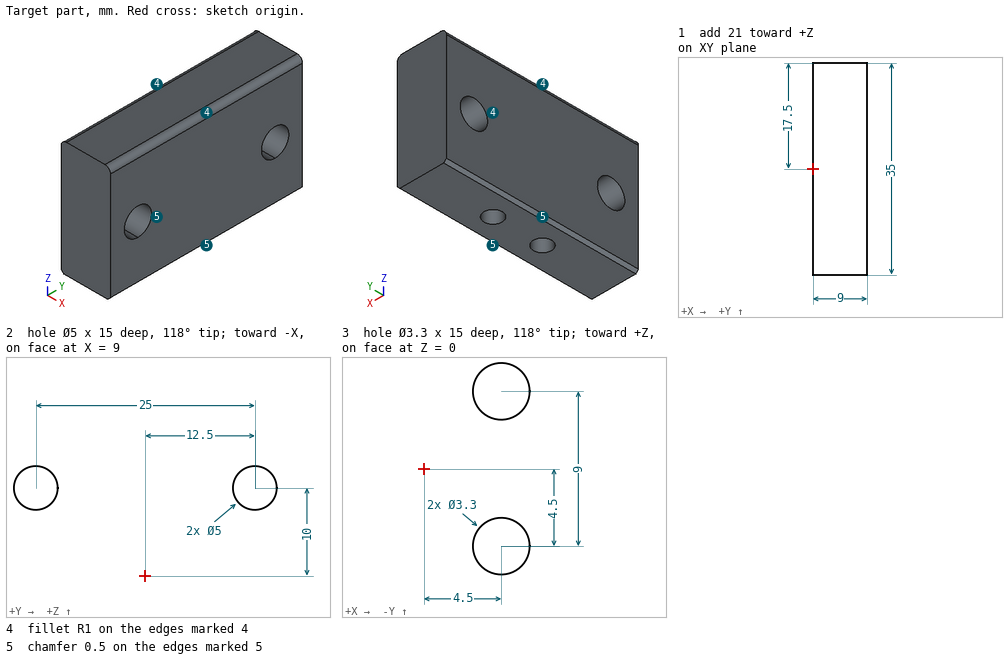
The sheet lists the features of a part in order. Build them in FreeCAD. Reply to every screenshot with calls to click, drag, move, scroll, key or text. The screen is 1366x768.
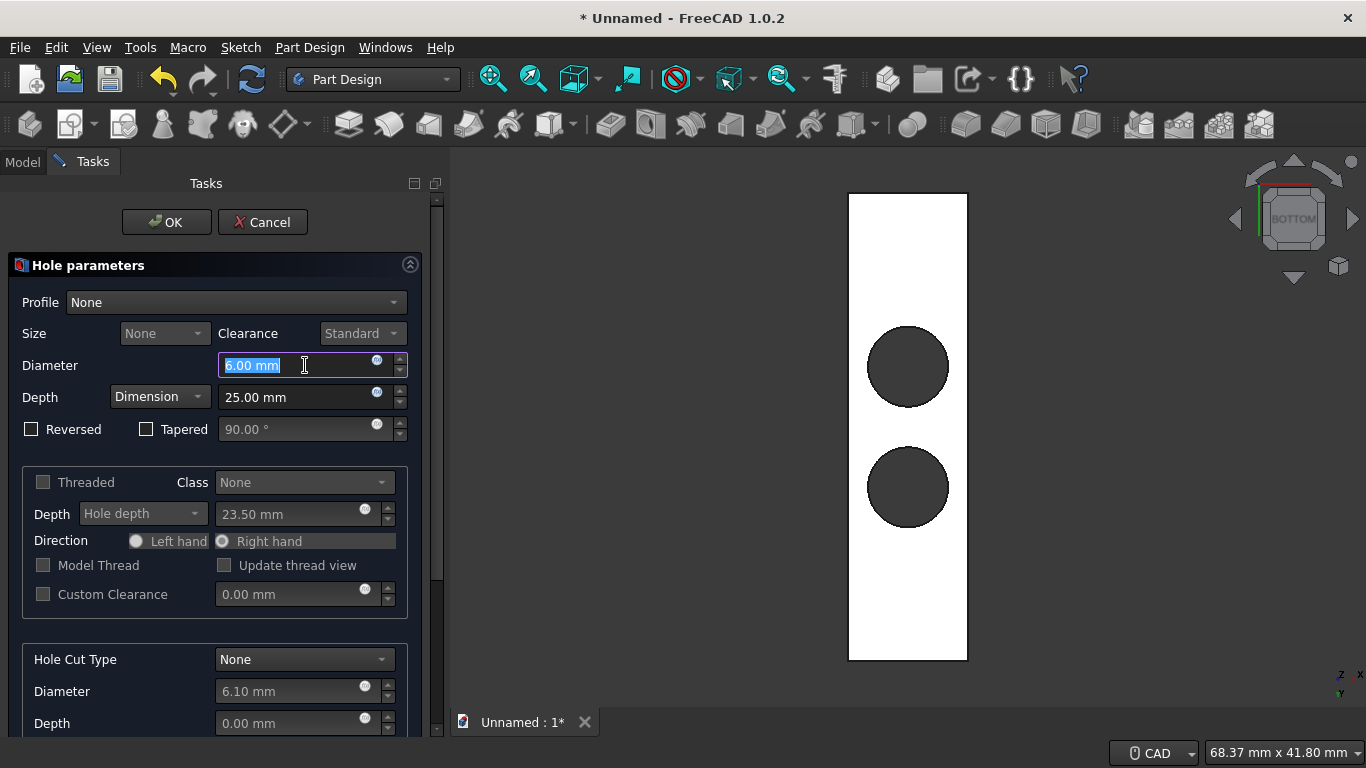
text(3.3)
key(Tab)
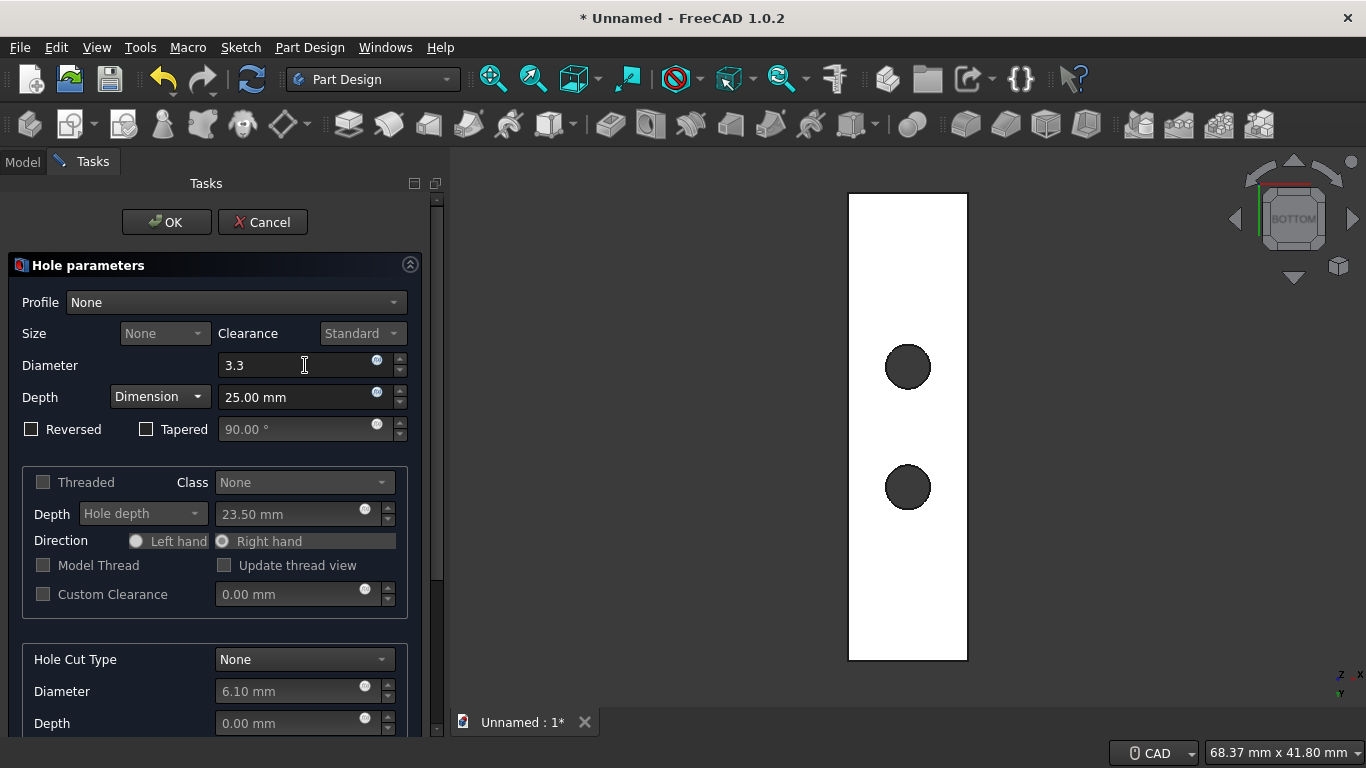
triple_click(305, 397)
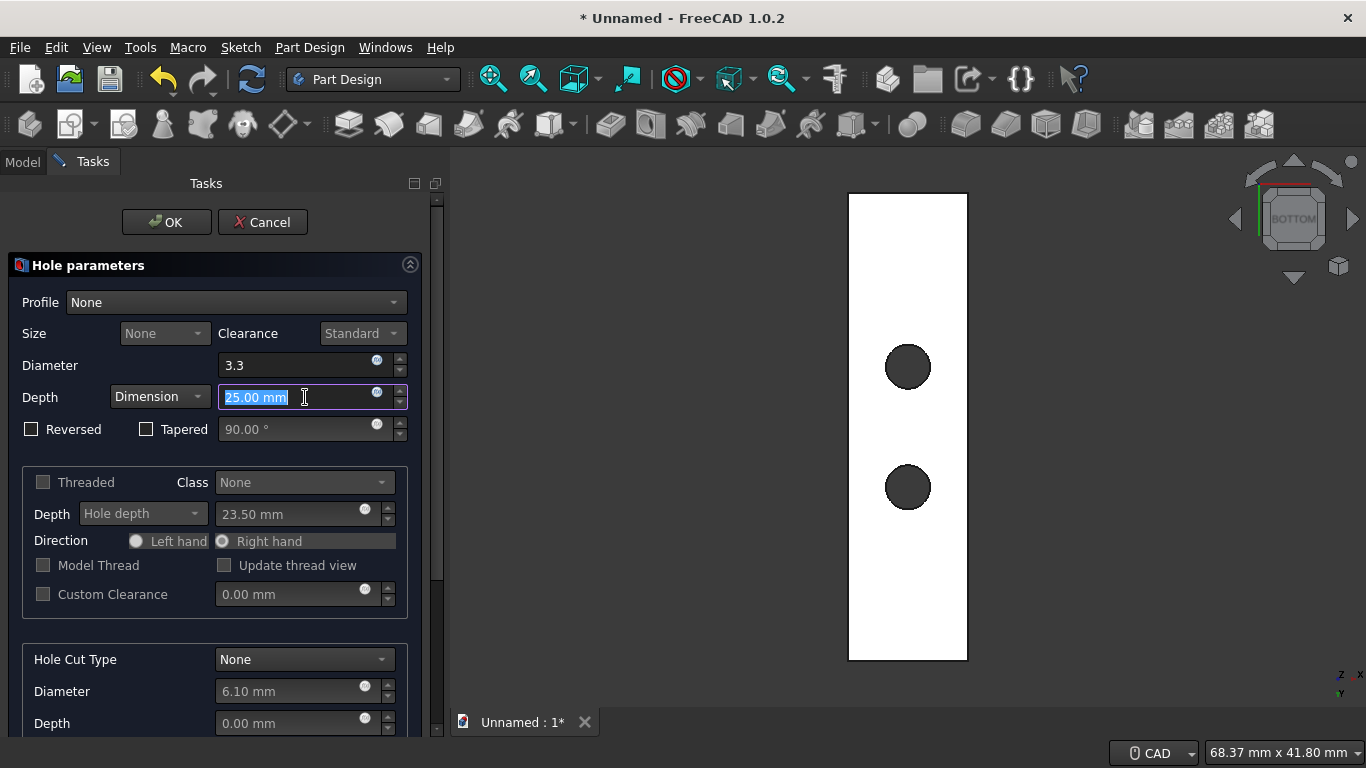
text(15)
key(Tab)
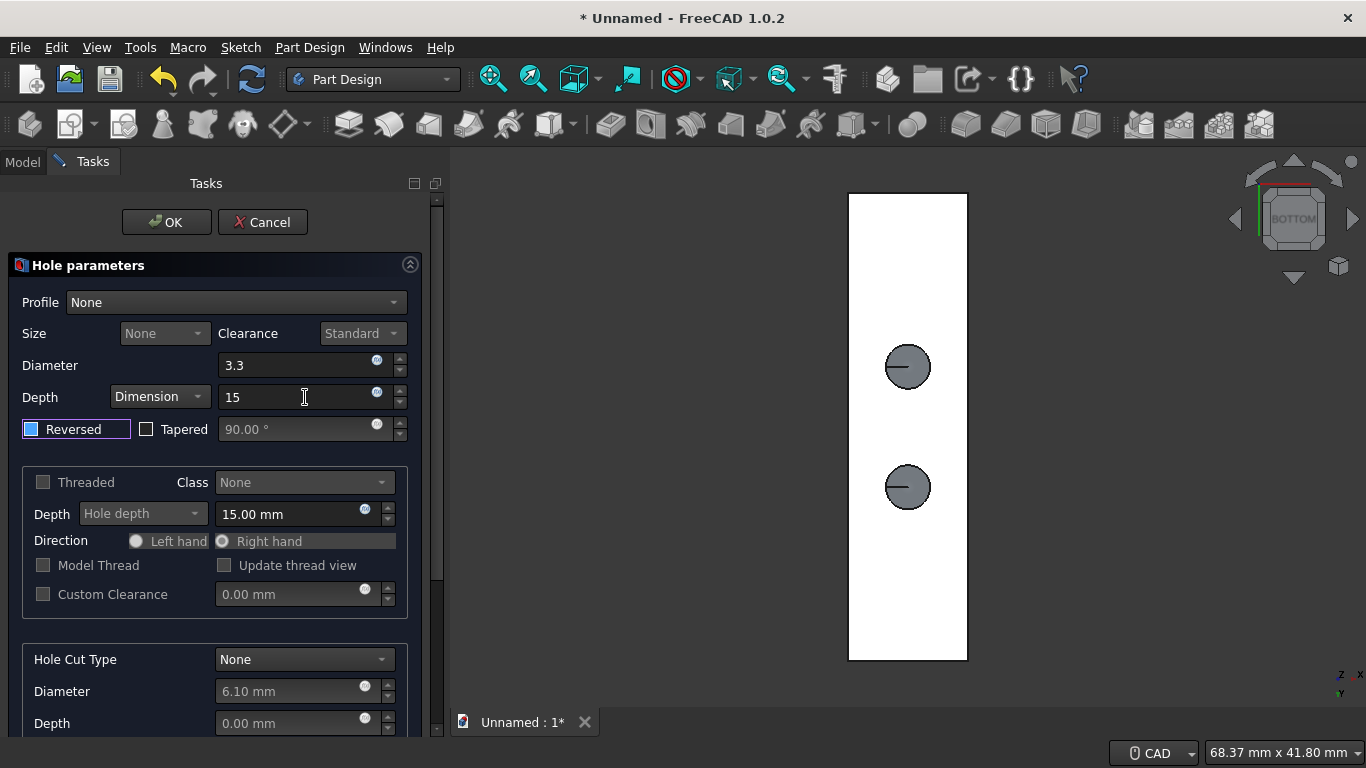
click(167, 222)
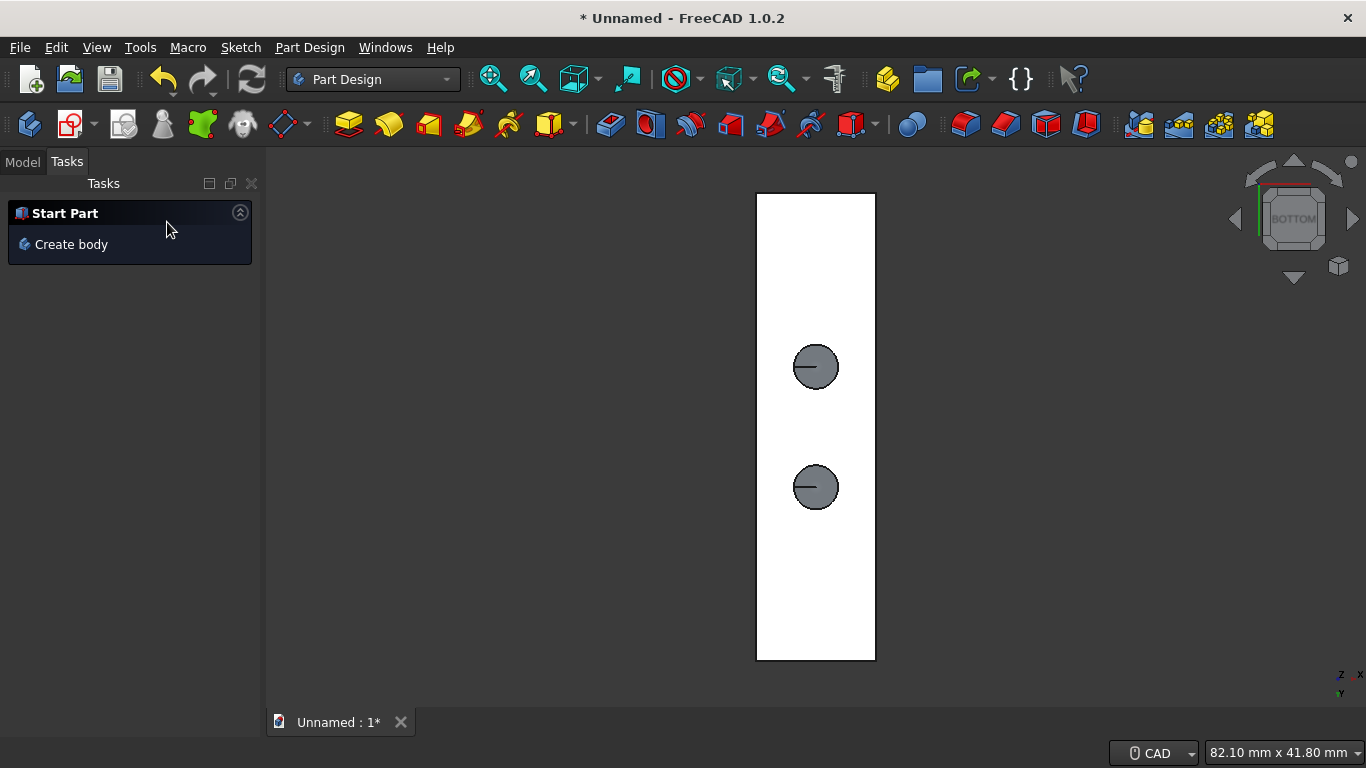
key(0)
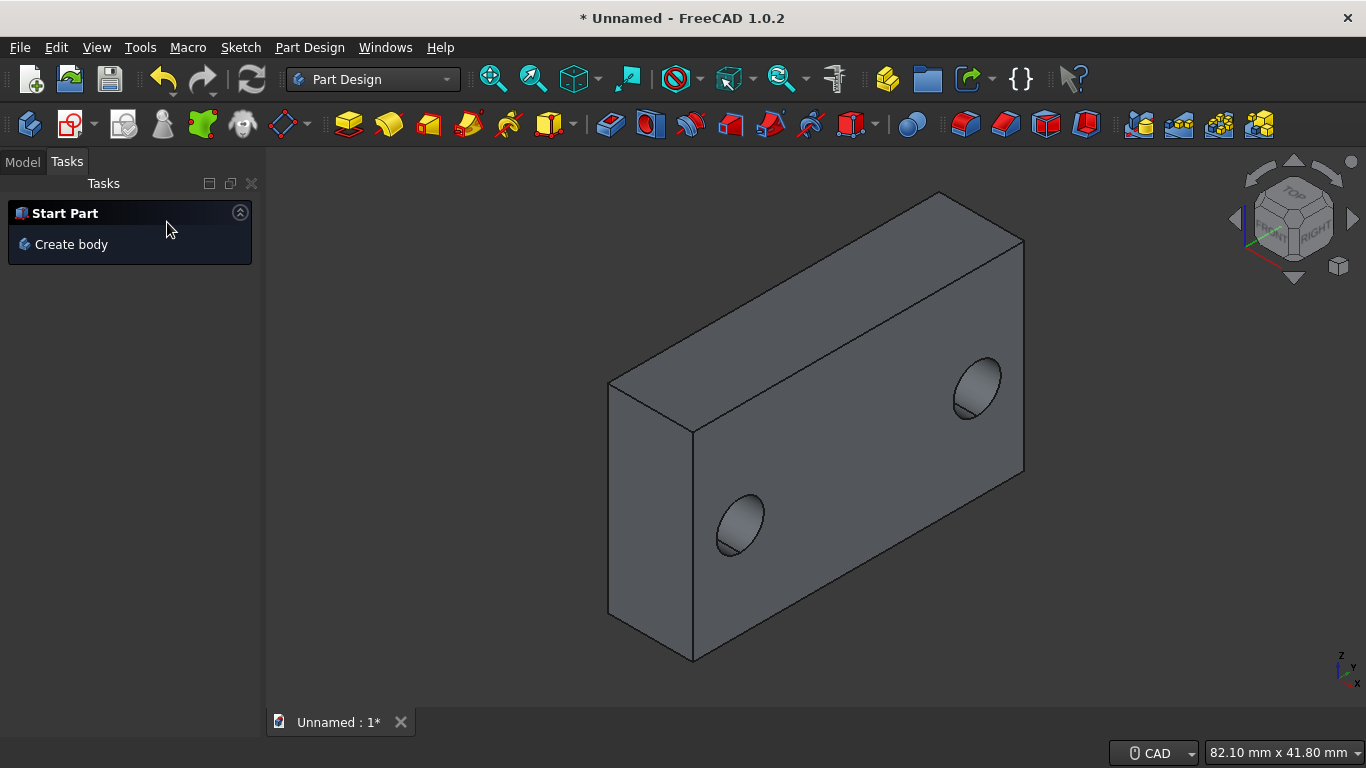
click(859, 336)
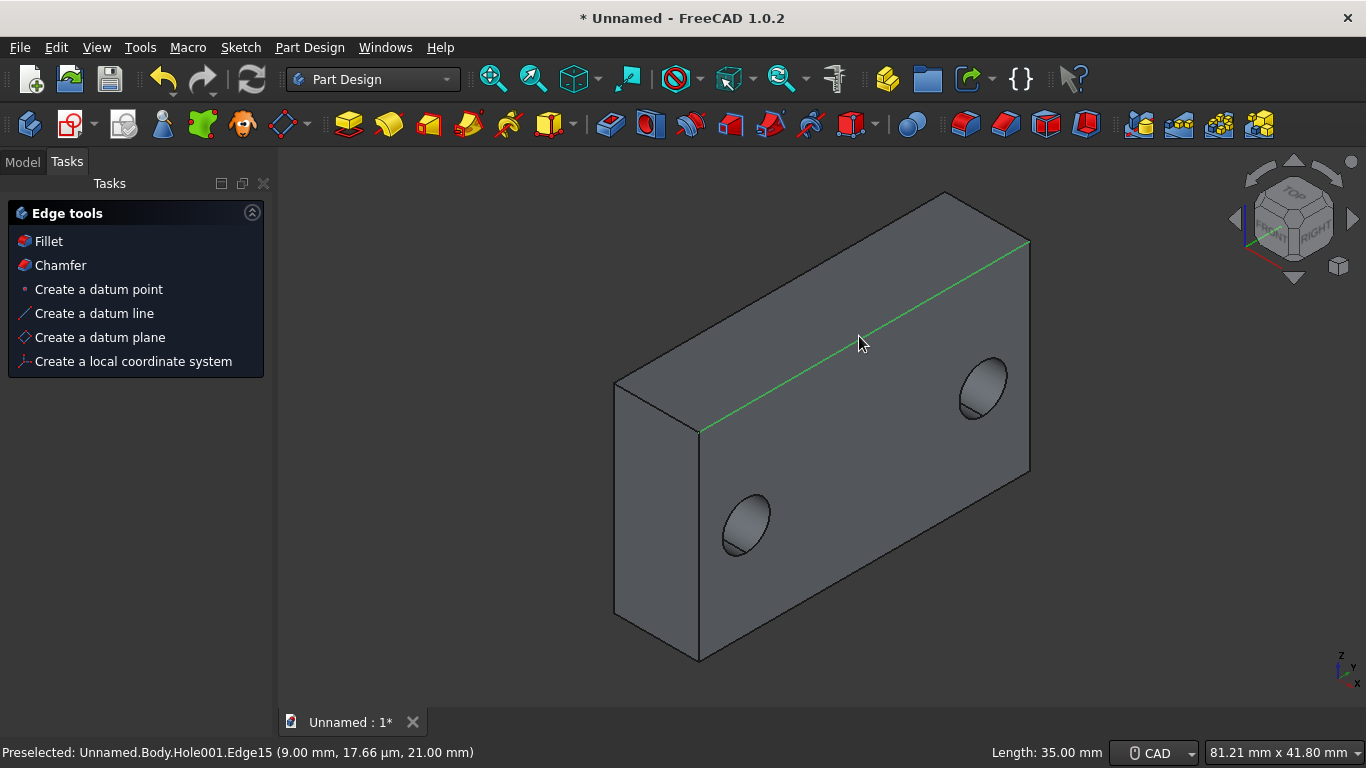
key(2)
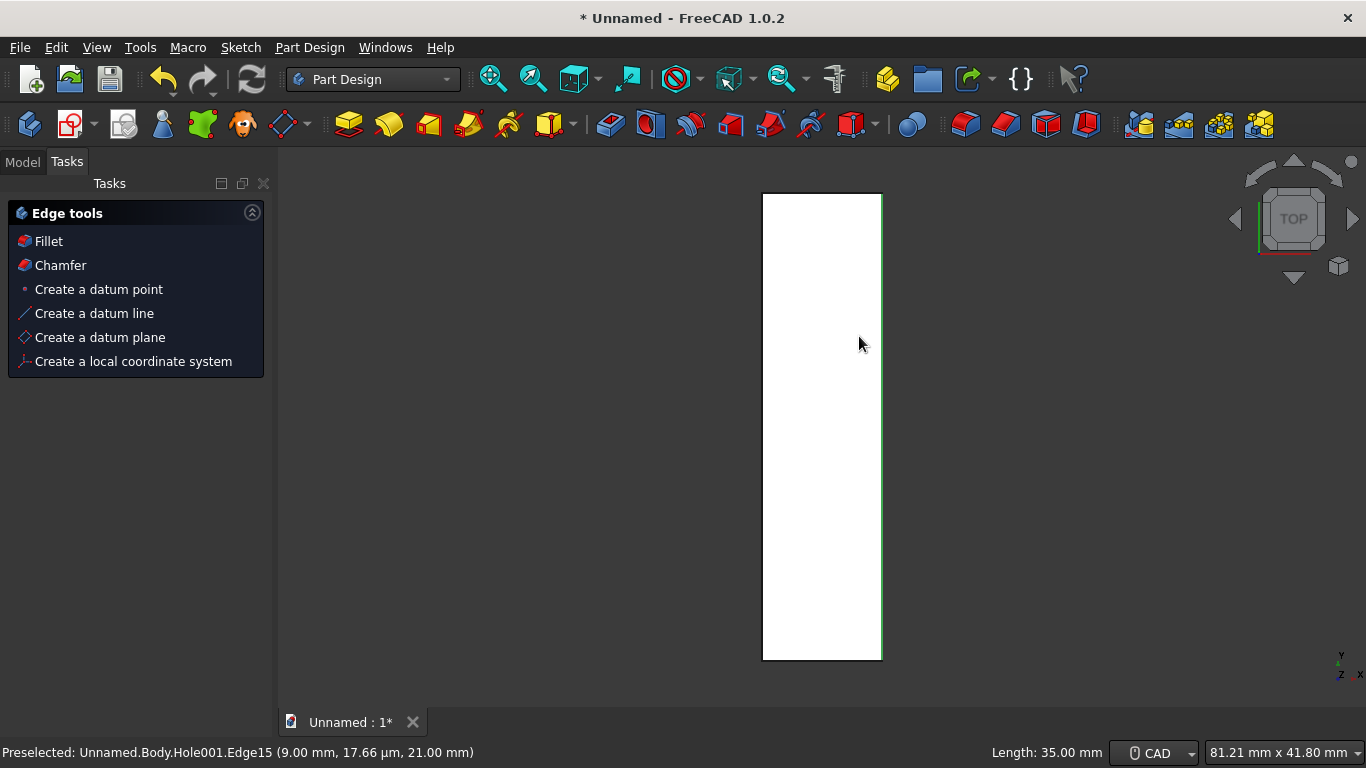
click(762, 426, ctrl)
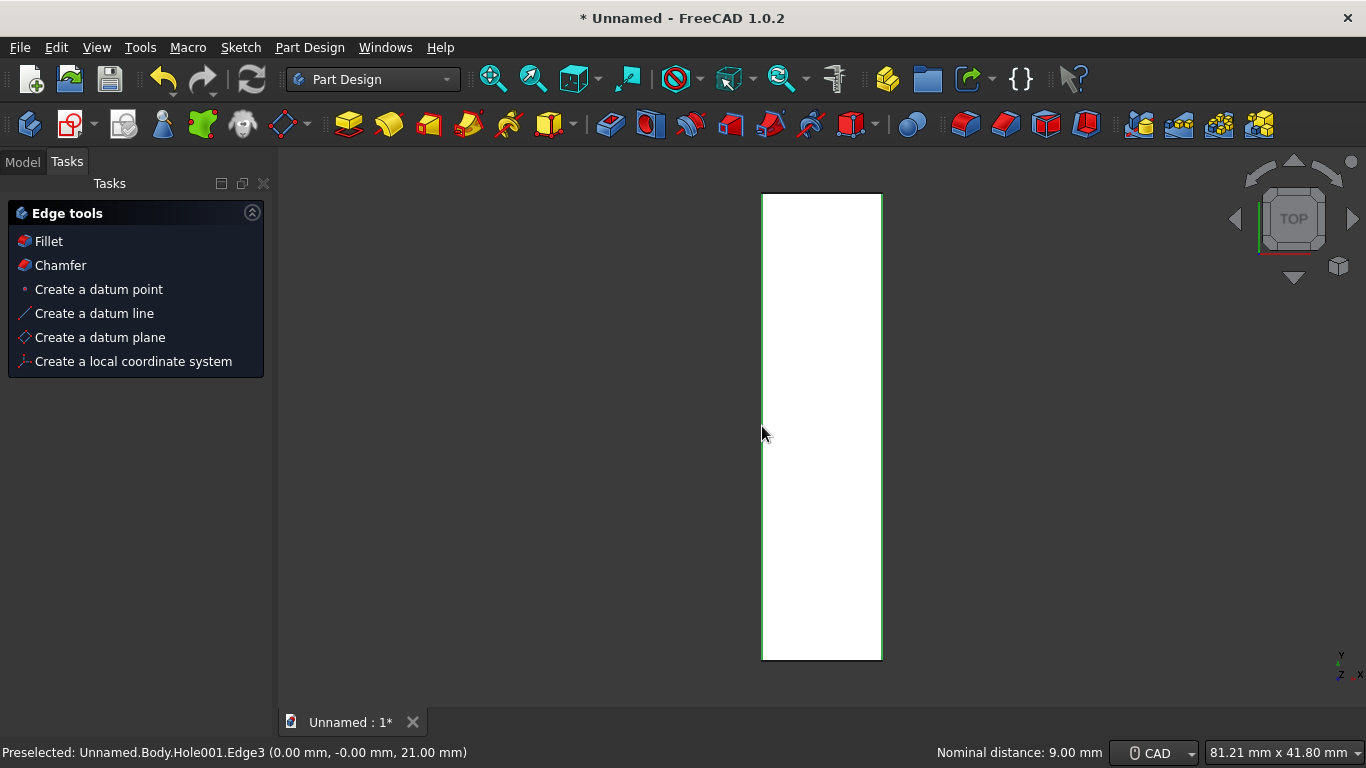
click(966, 124)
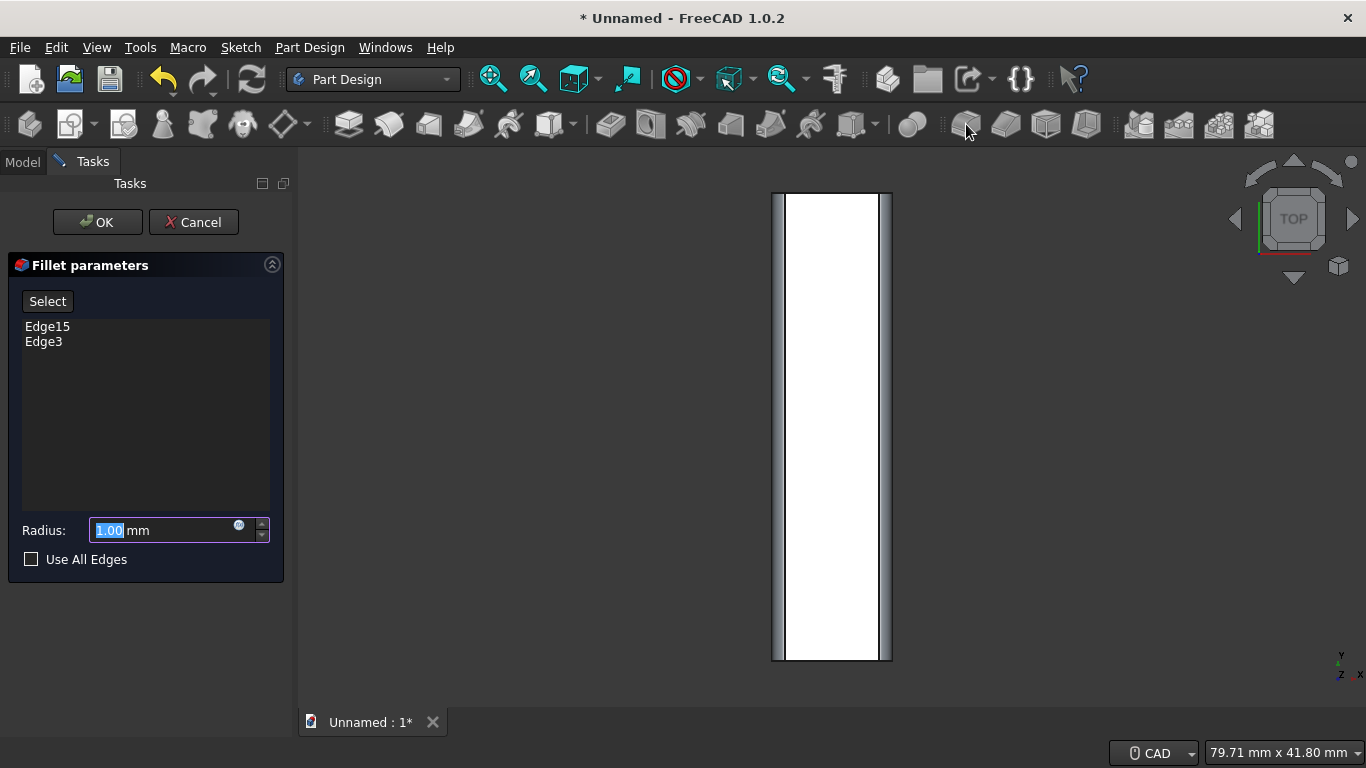
text(1)
key(Tab)